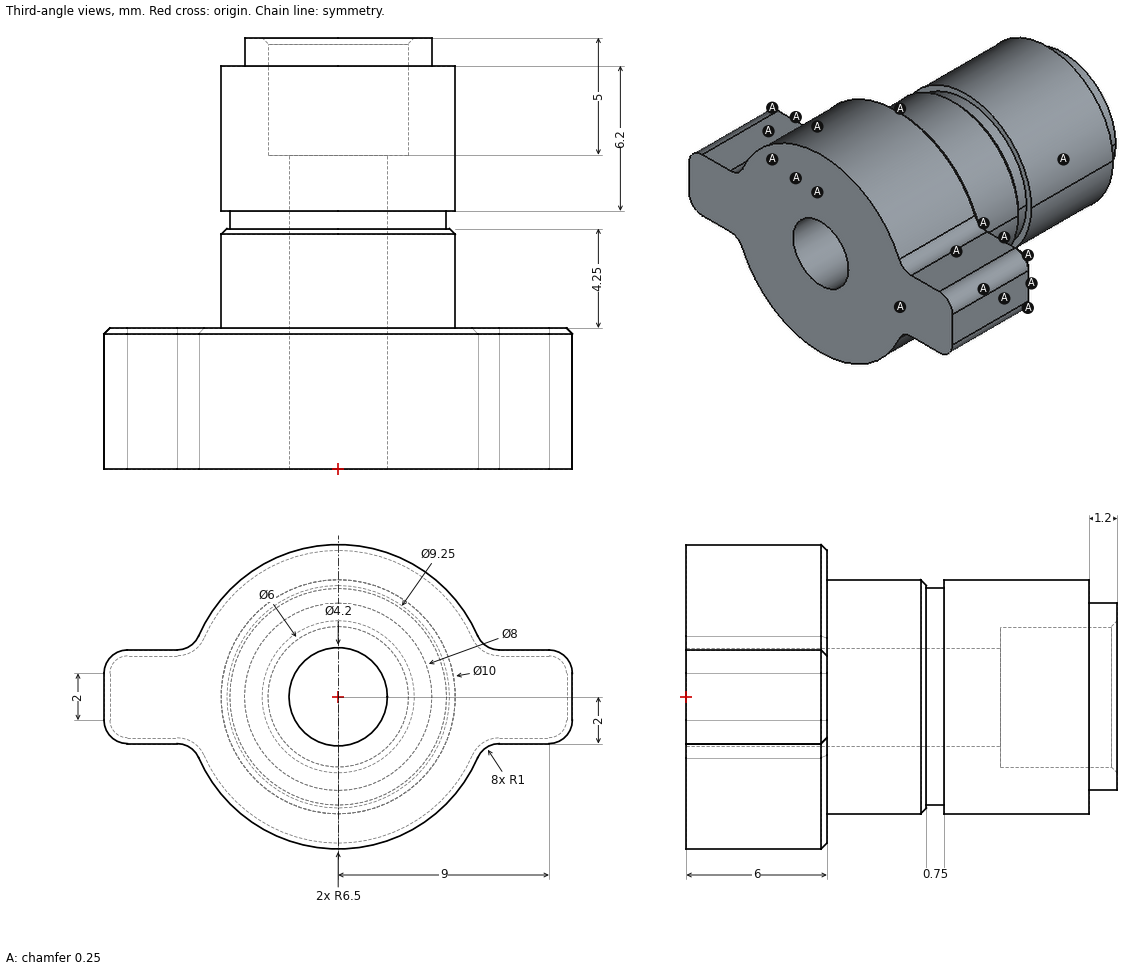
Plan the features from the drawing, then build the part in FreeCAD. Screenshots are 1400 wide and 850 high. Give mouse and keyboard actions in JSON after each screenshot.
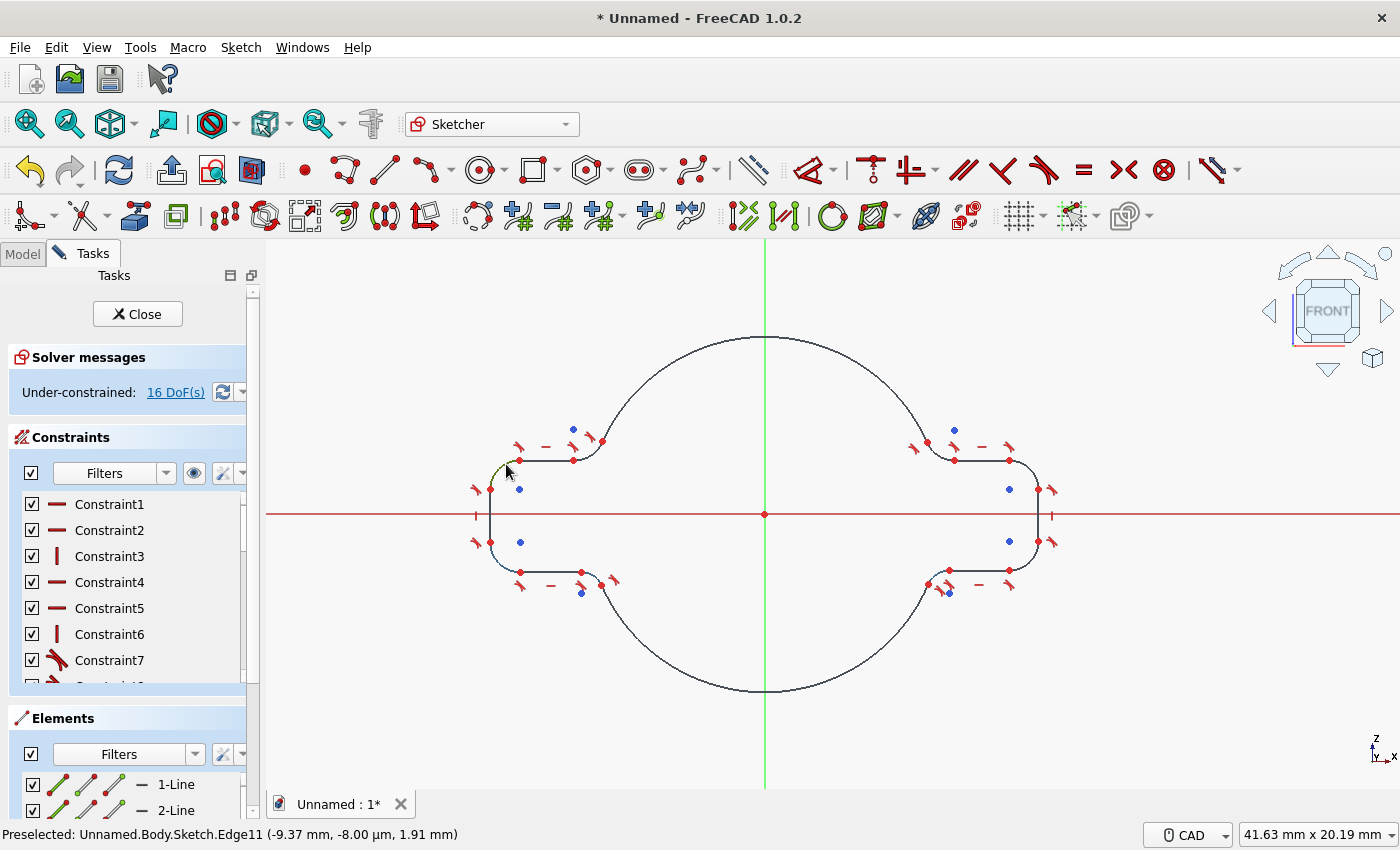
{"action": "scroll", "coordinate": [584, 459], "scroll_direction": "up", "scroll_amount": 2}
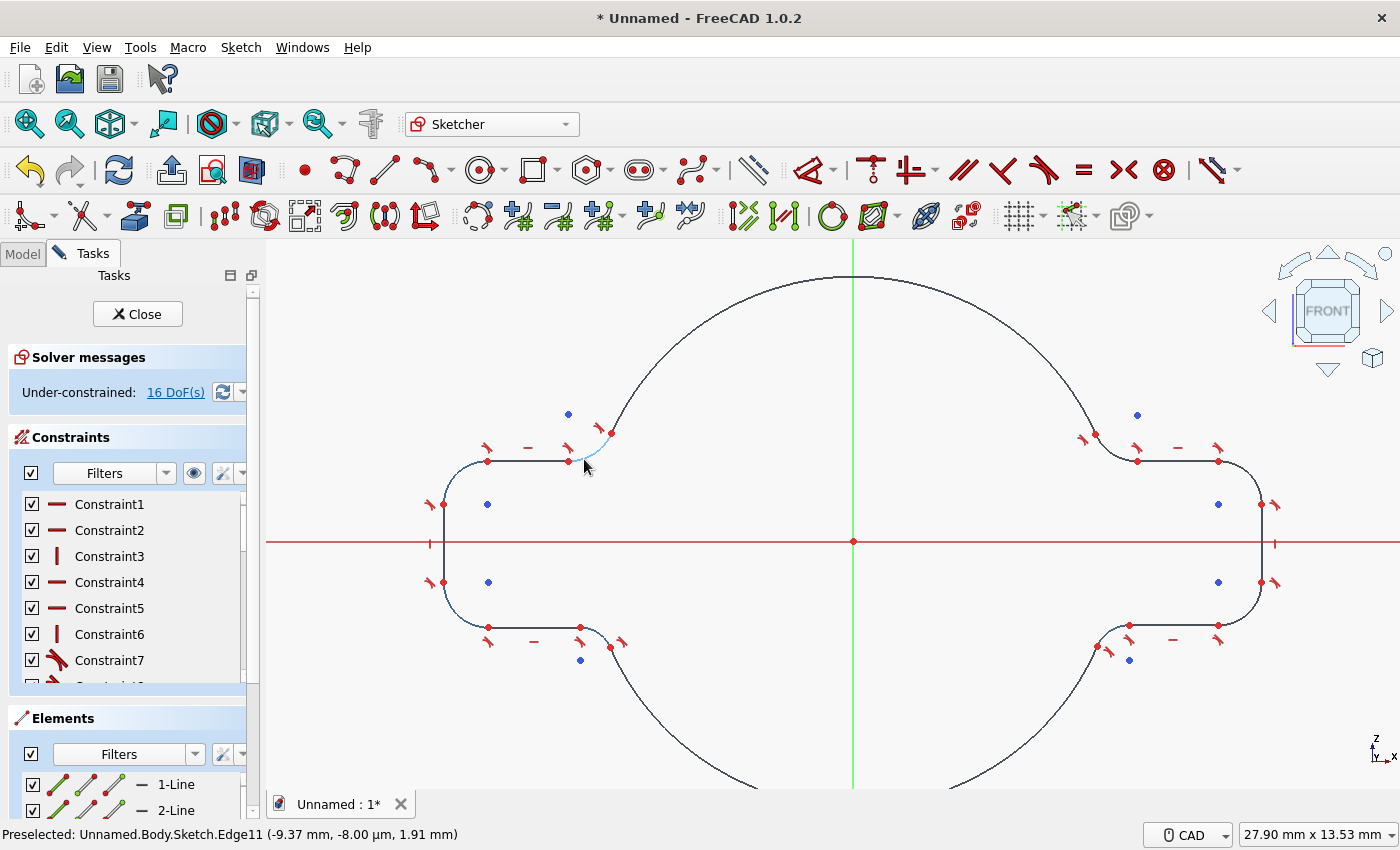
{"action": "left_click", "coordinate": [585, 459]}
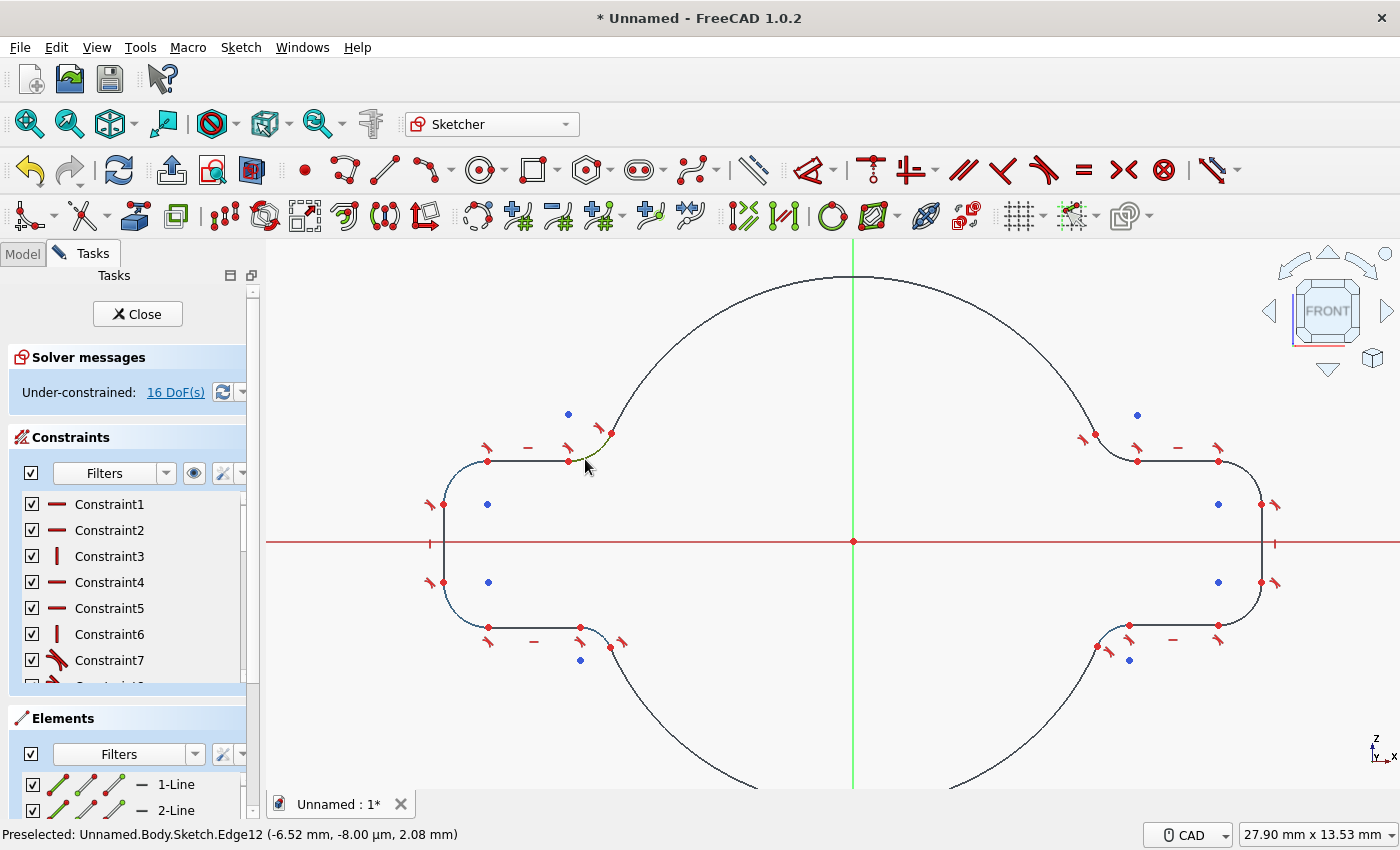
{"action": "left_click", "coordinate": [1104, 447]}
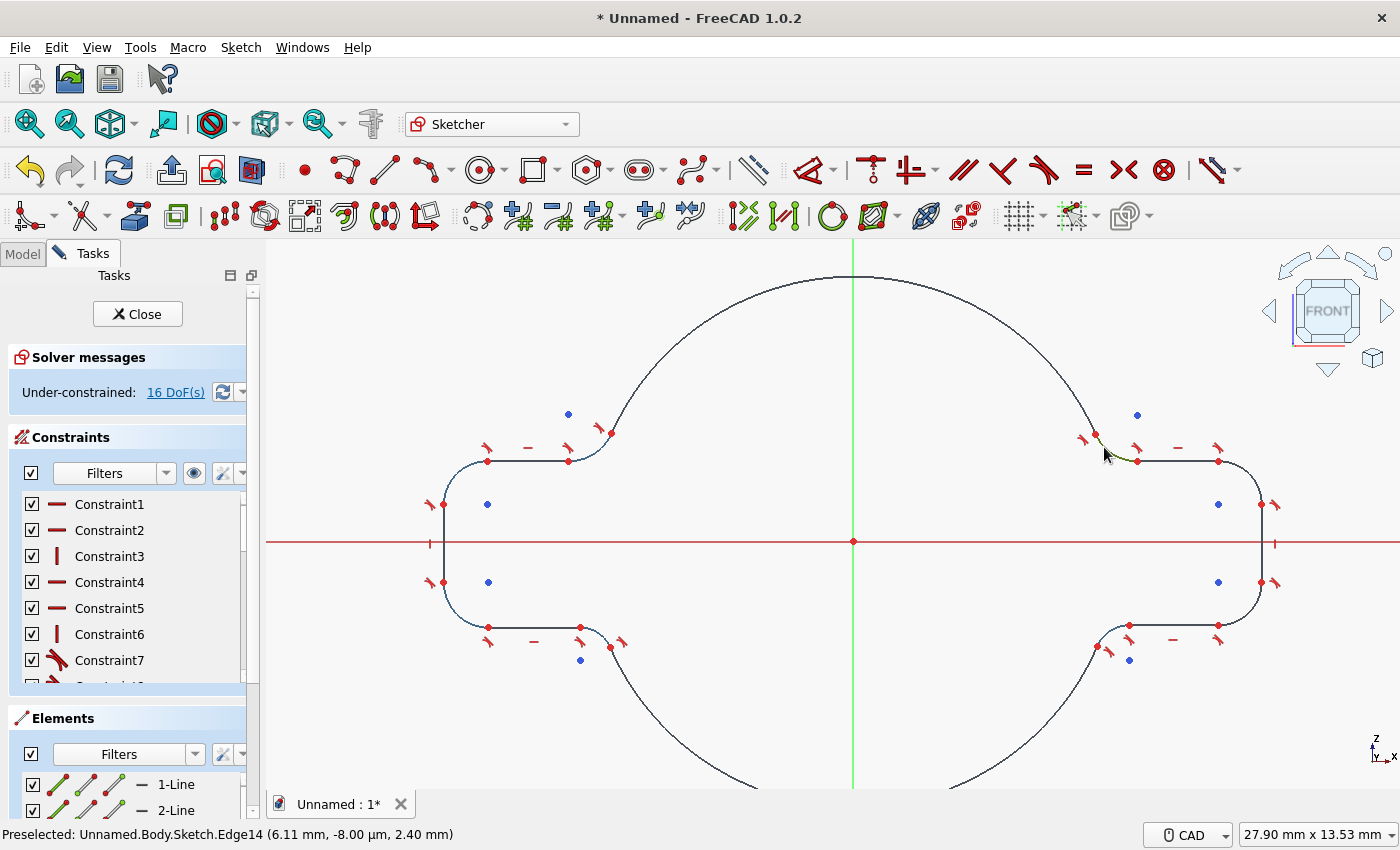
{"action": "left_click", "coordinate": [1232, 463]}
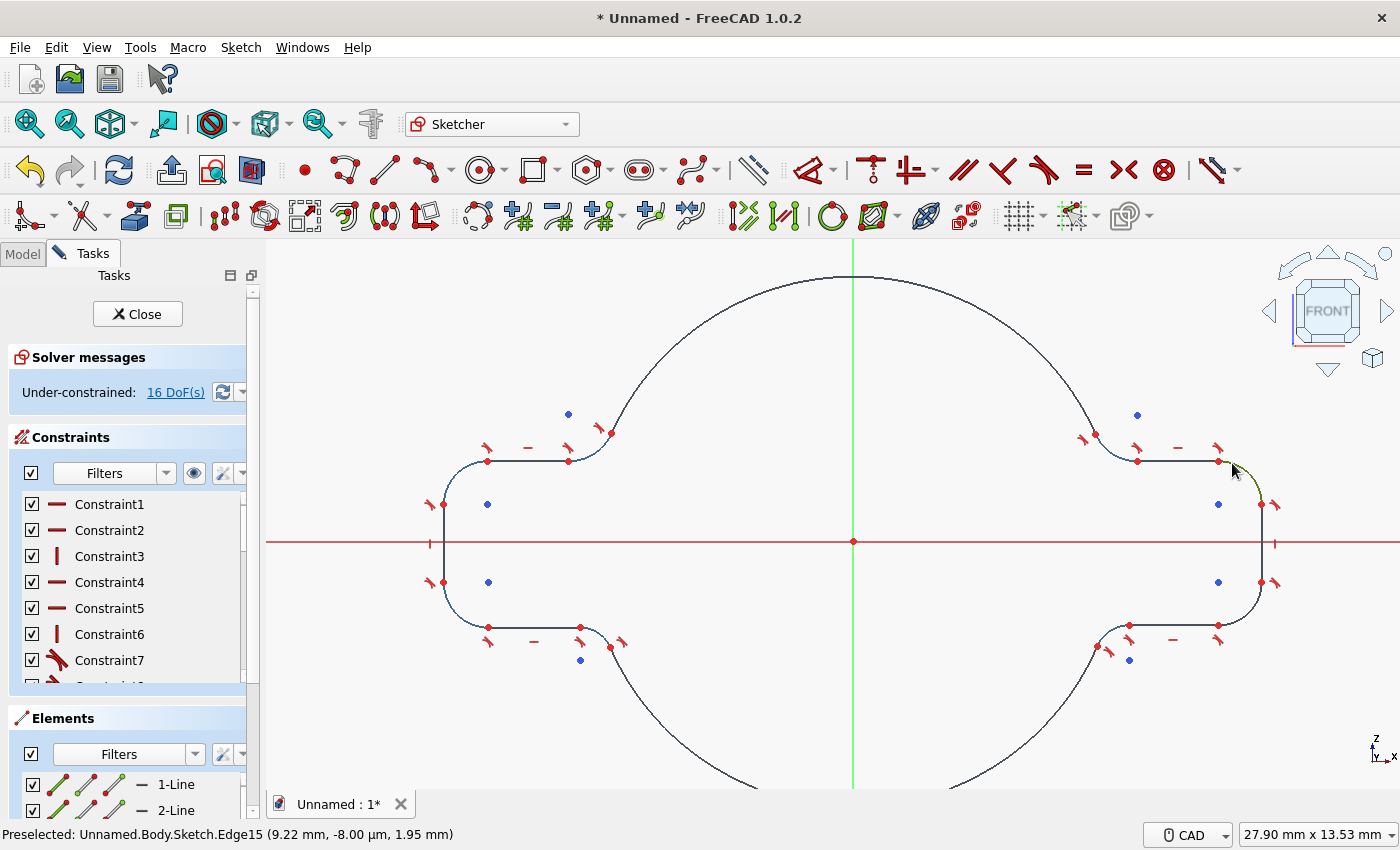
{"action": "left_click", "coordinate": [1232, 623]}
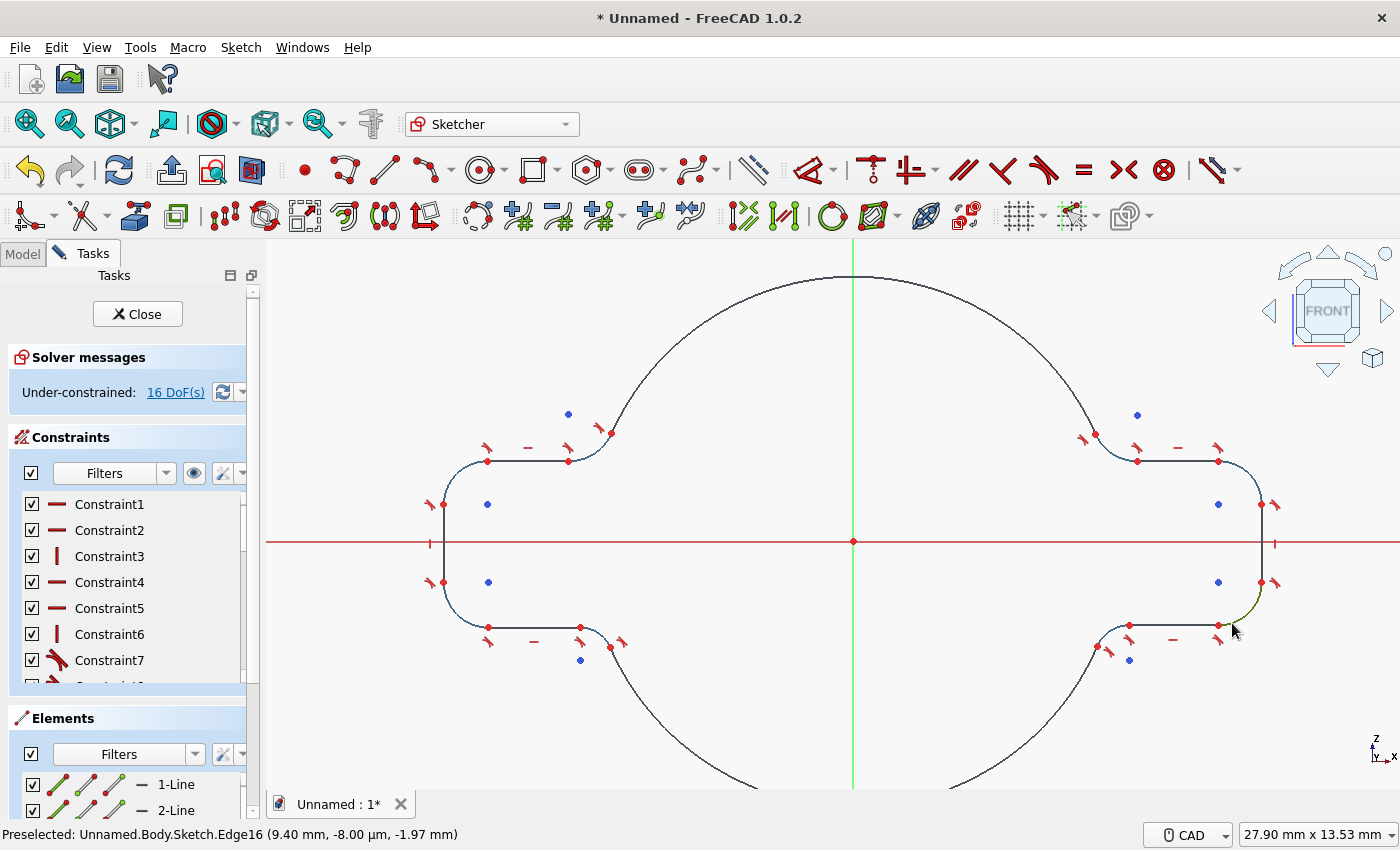
{"action": "left_click", "coordinate": [1084, 170]}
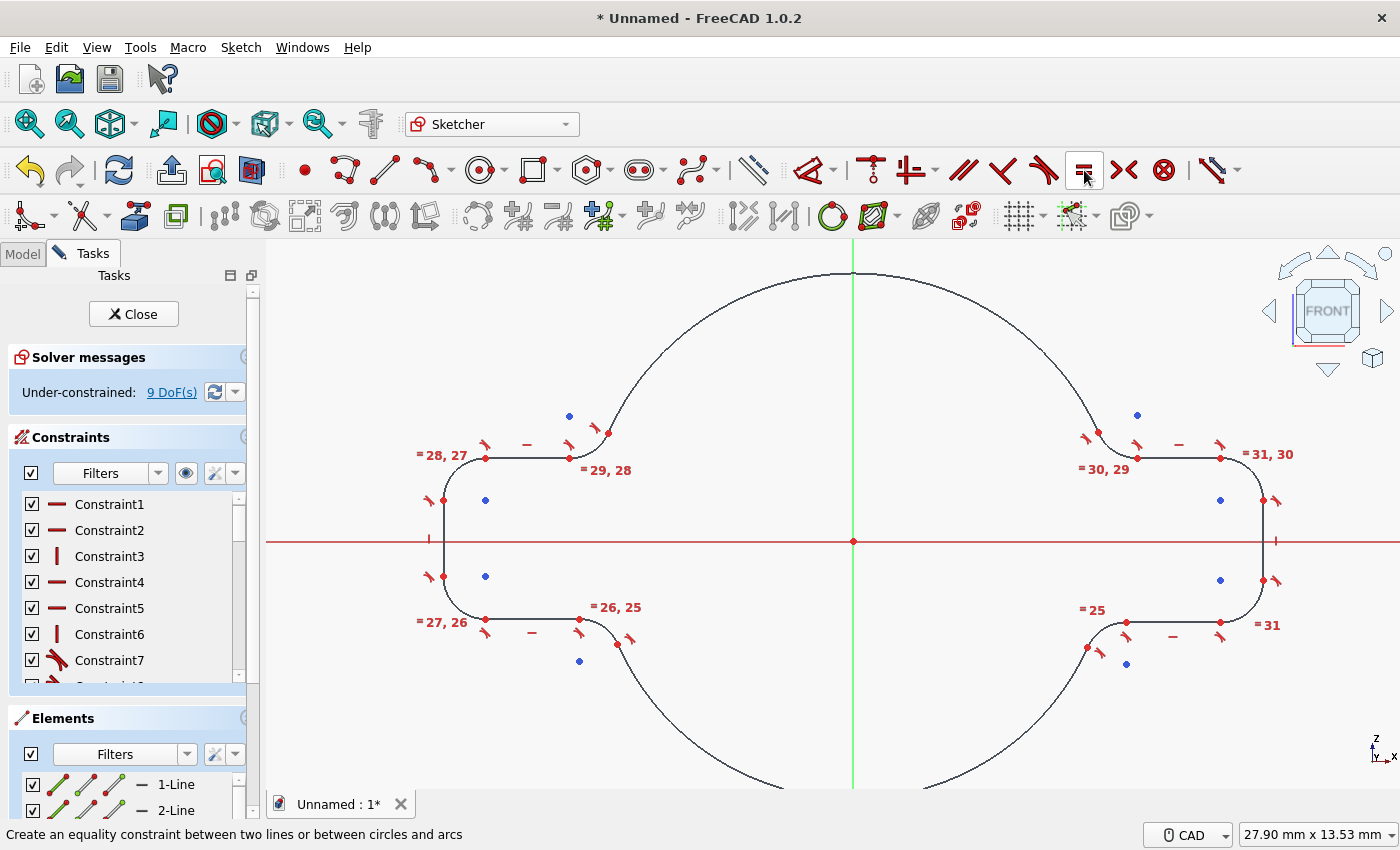
{"action": "left_click", "coordinate": [688, 738]}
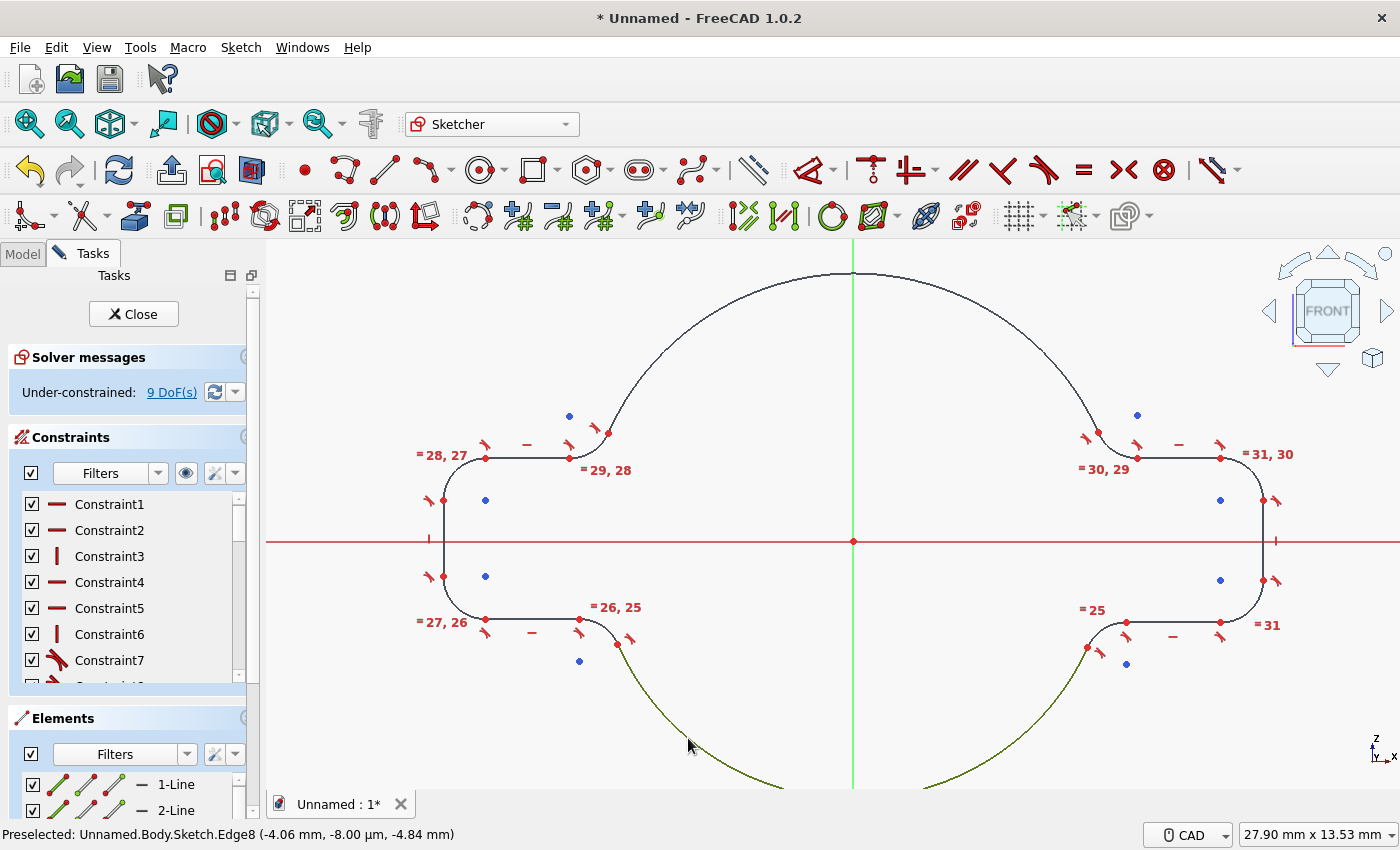
{"action": "left_click", "coordinate": [973, 301]}